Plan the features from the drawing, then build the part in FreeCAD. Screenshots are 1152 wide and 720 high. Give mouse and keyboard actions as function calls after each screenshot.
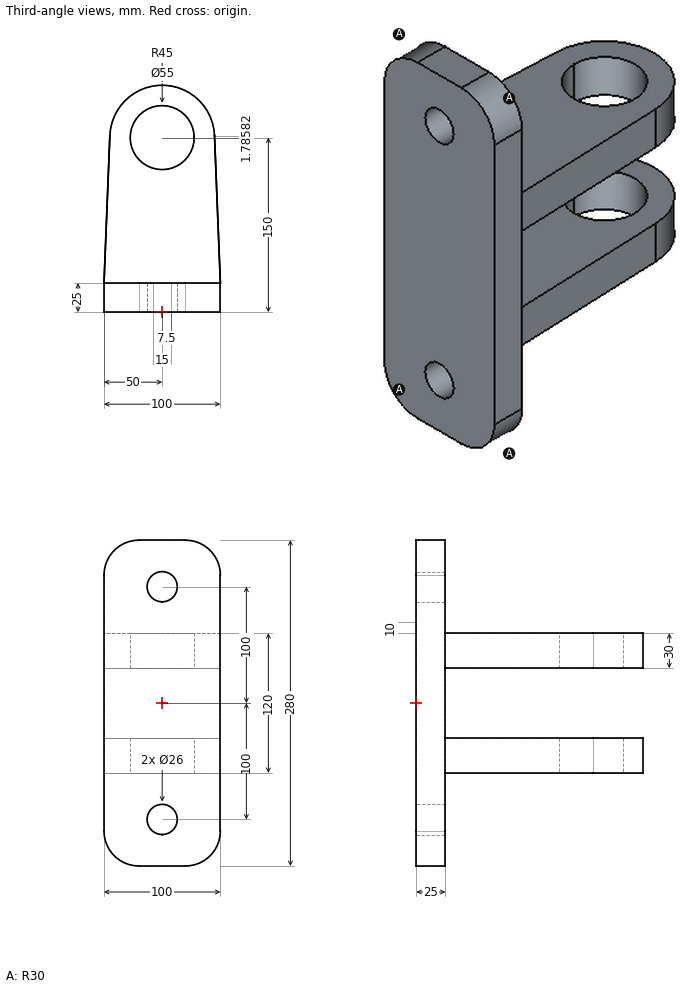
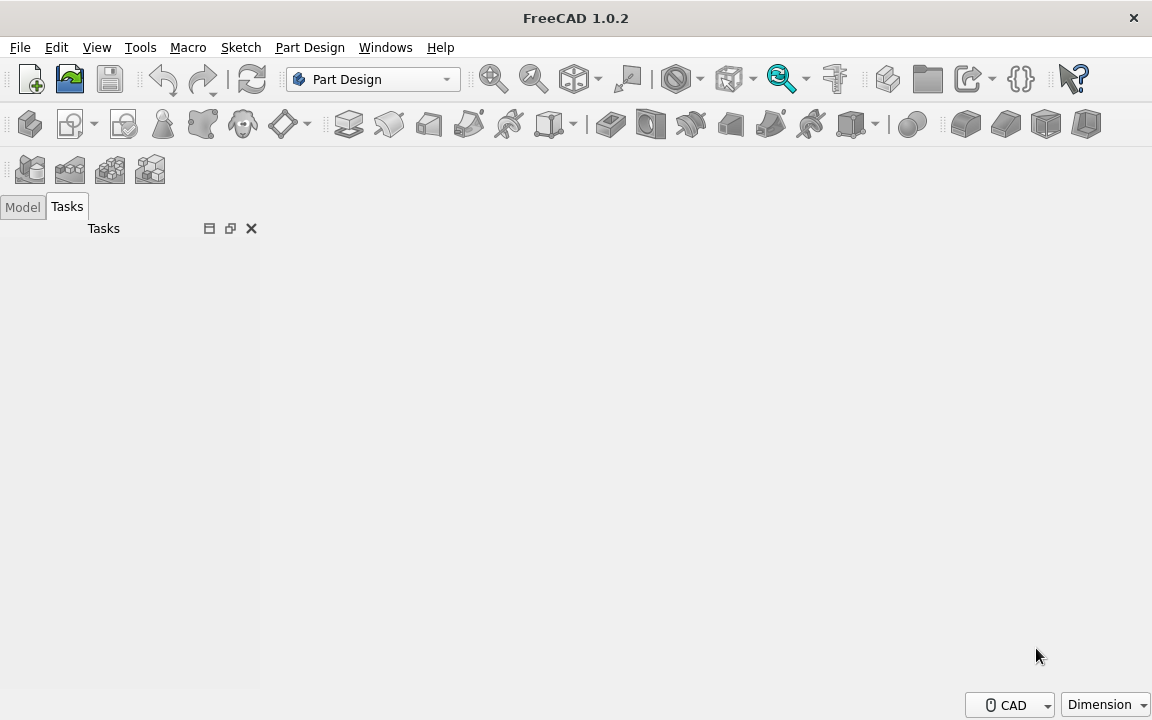
click(30, 80)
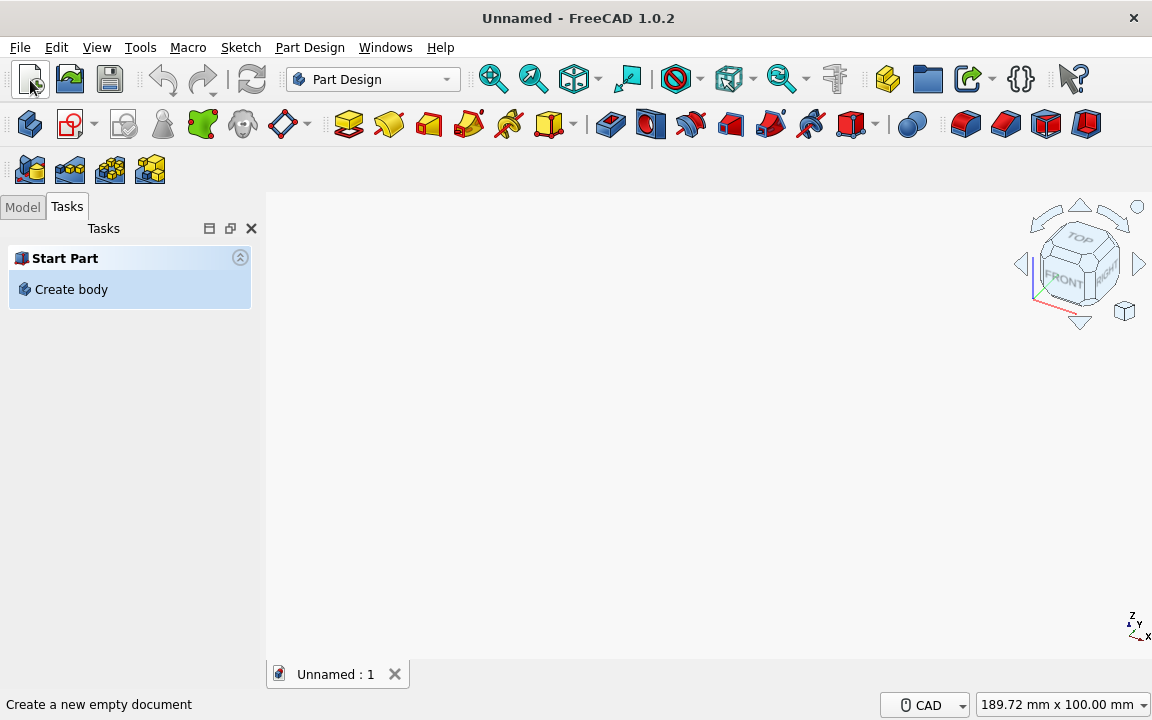
click(70, 124)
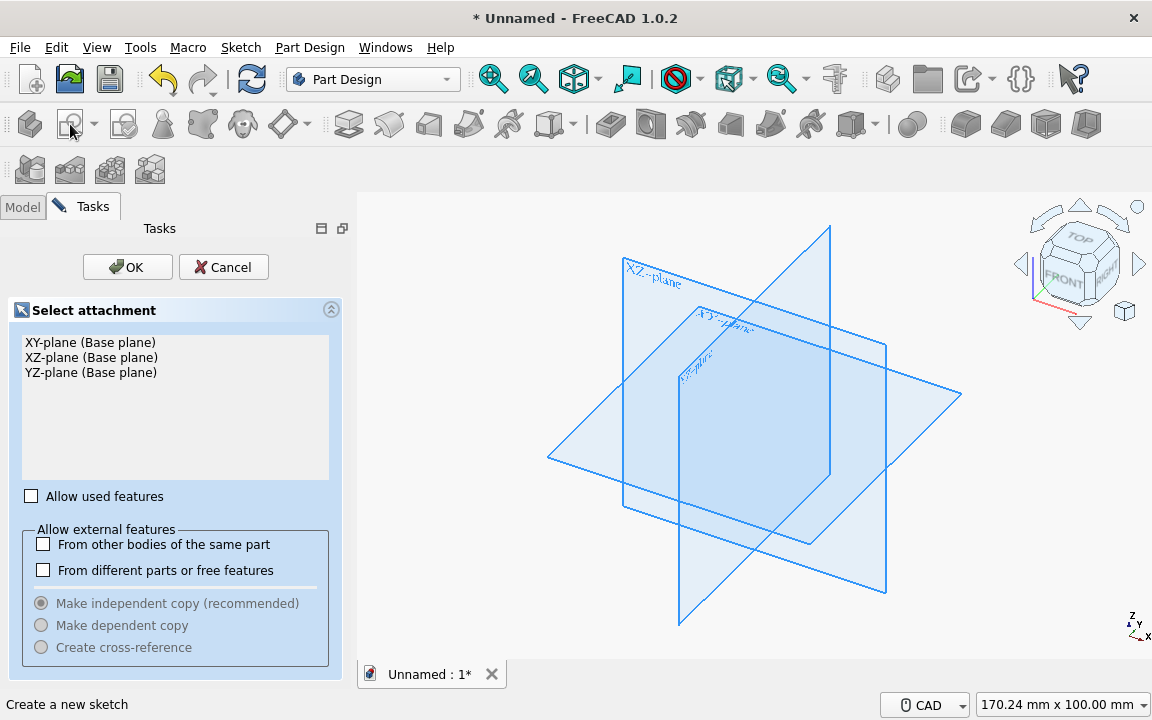
click(82, 358)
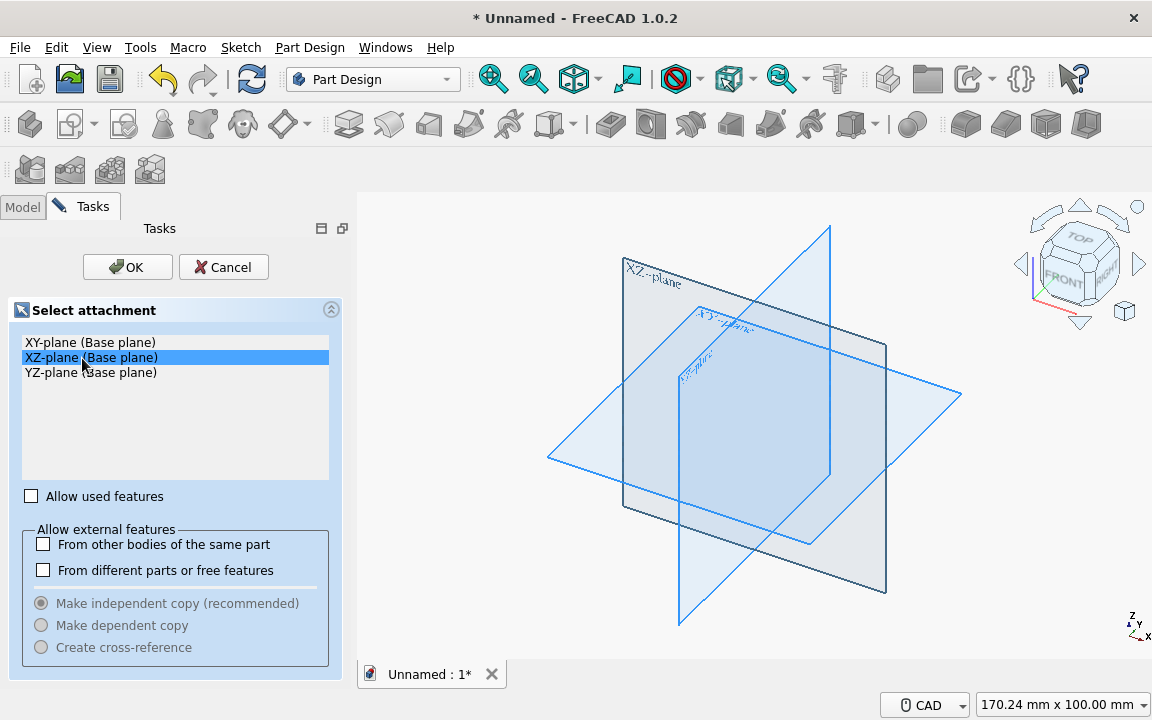
click(128, 267)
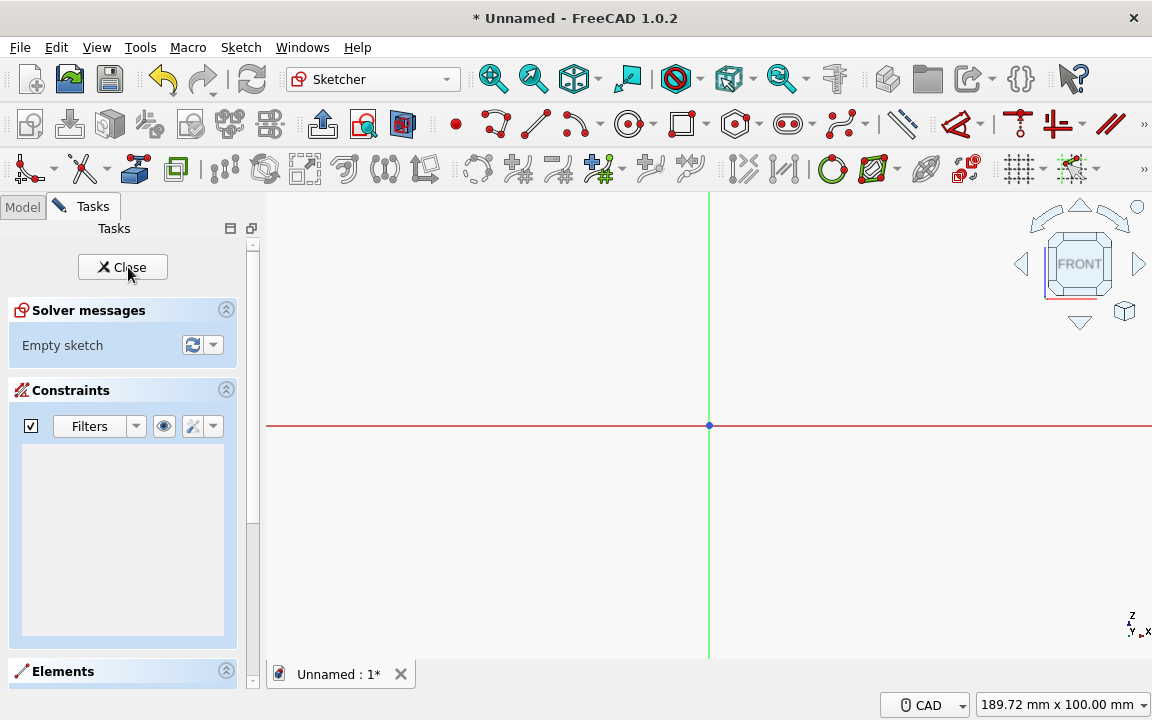
scroll(557, 426, down, 3)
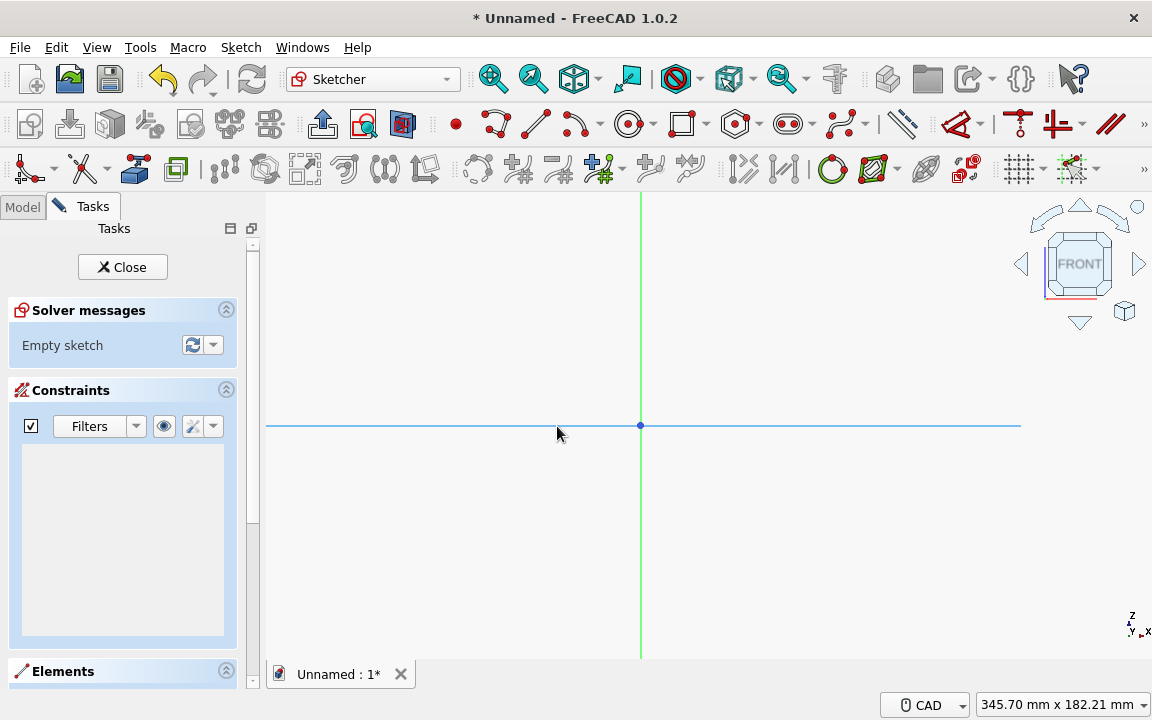
key(g)
key(v)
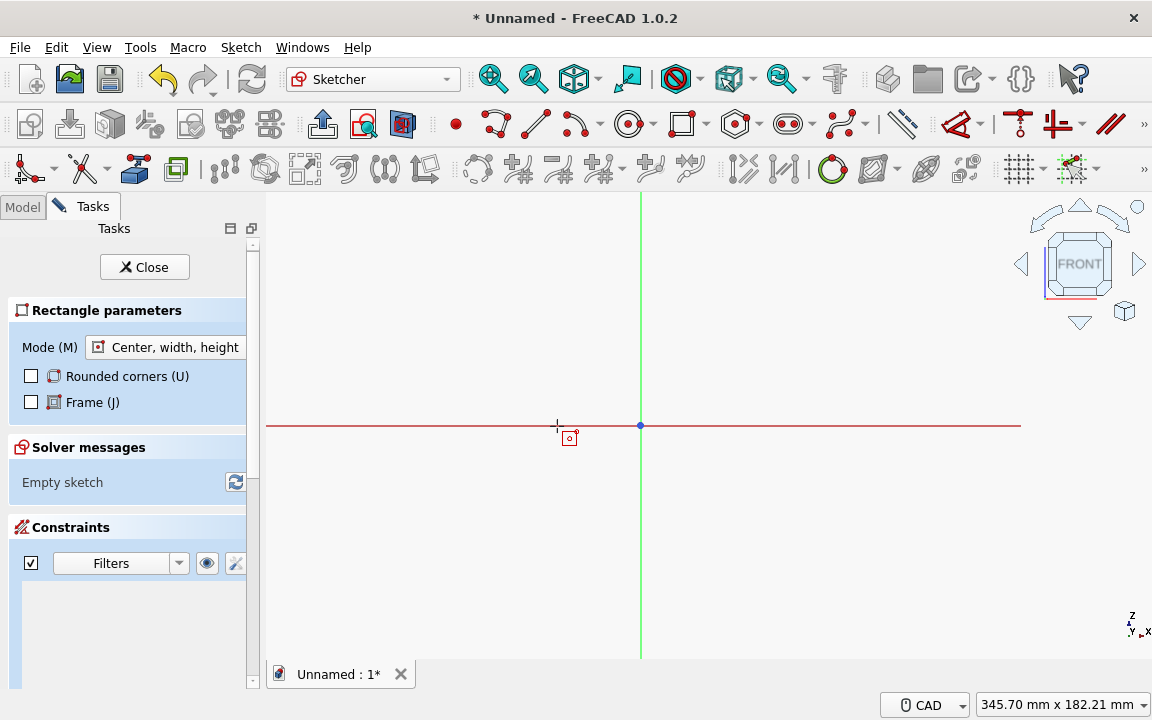
click(641, 426)
click(769, 272)
key(Escape)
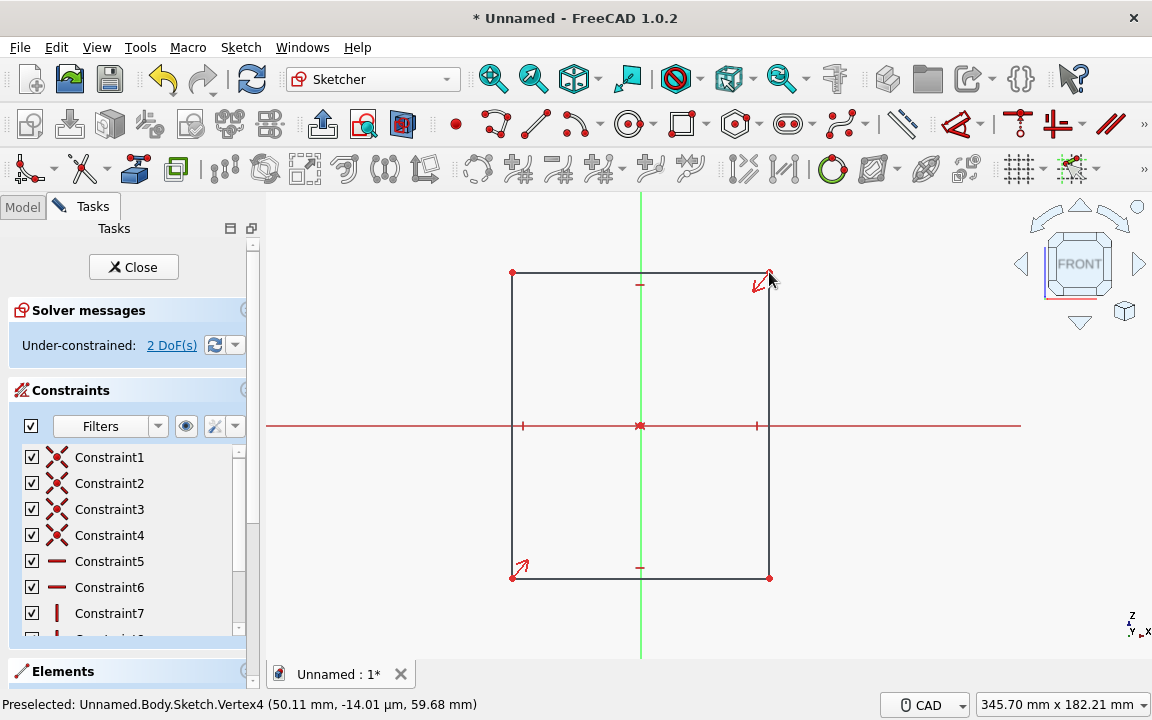
click(589, 579)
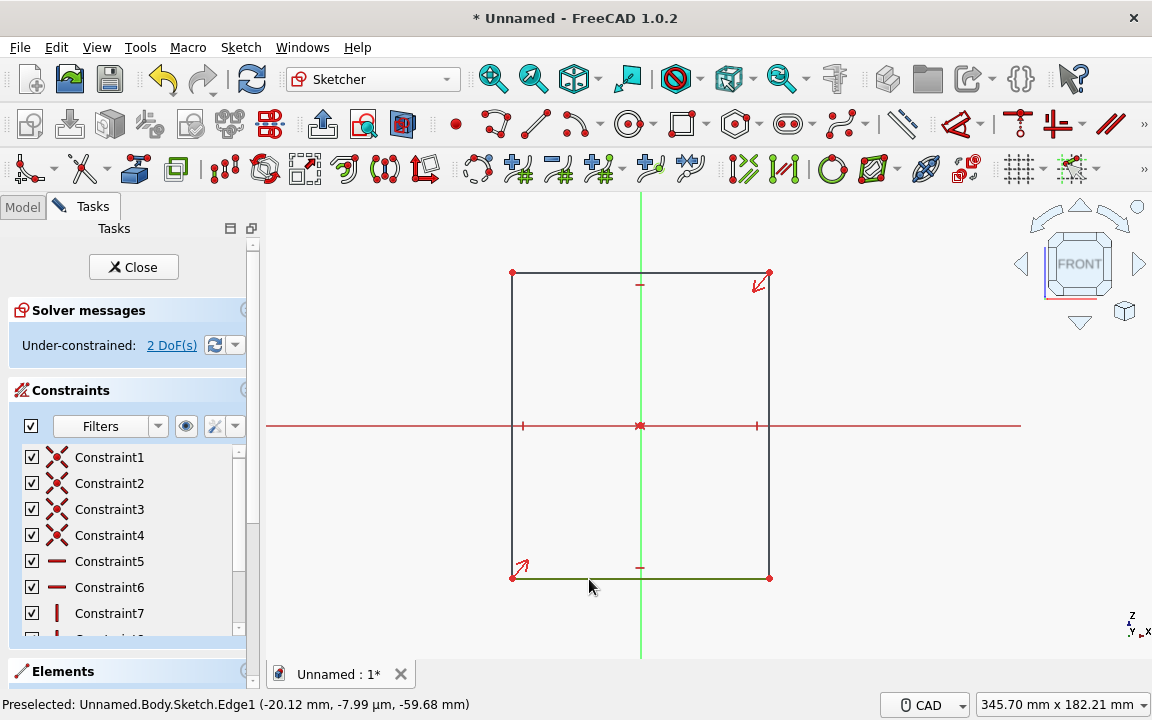
key(l)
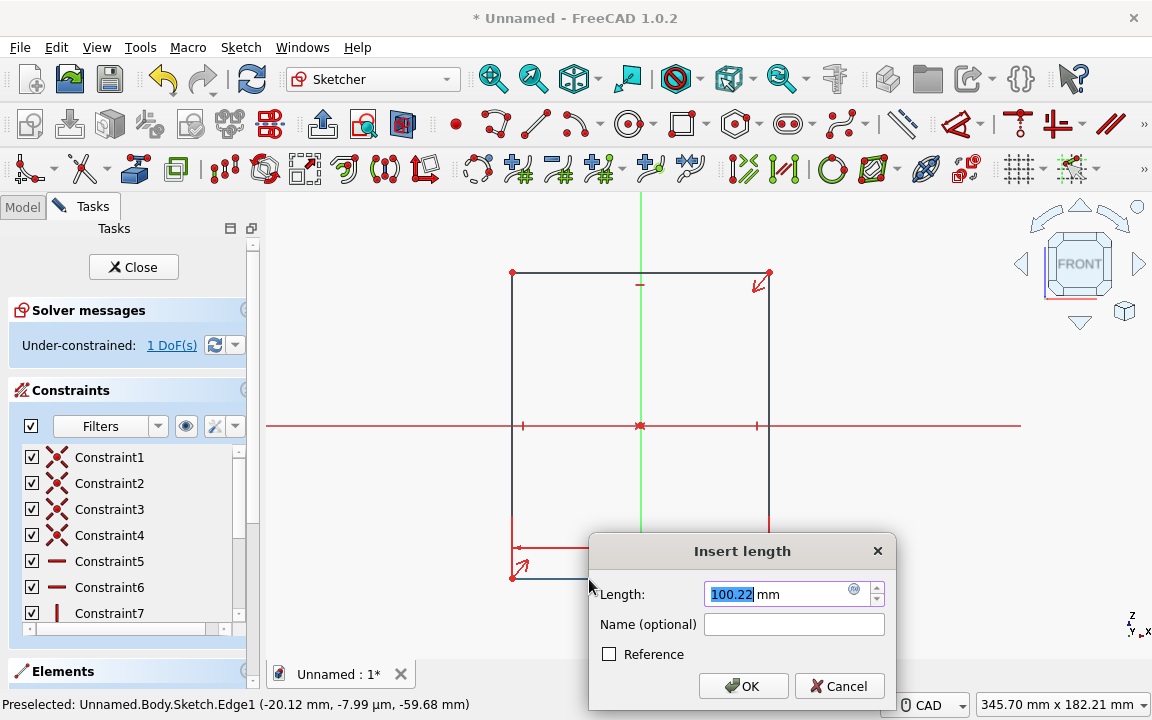
text(100)
key(Return)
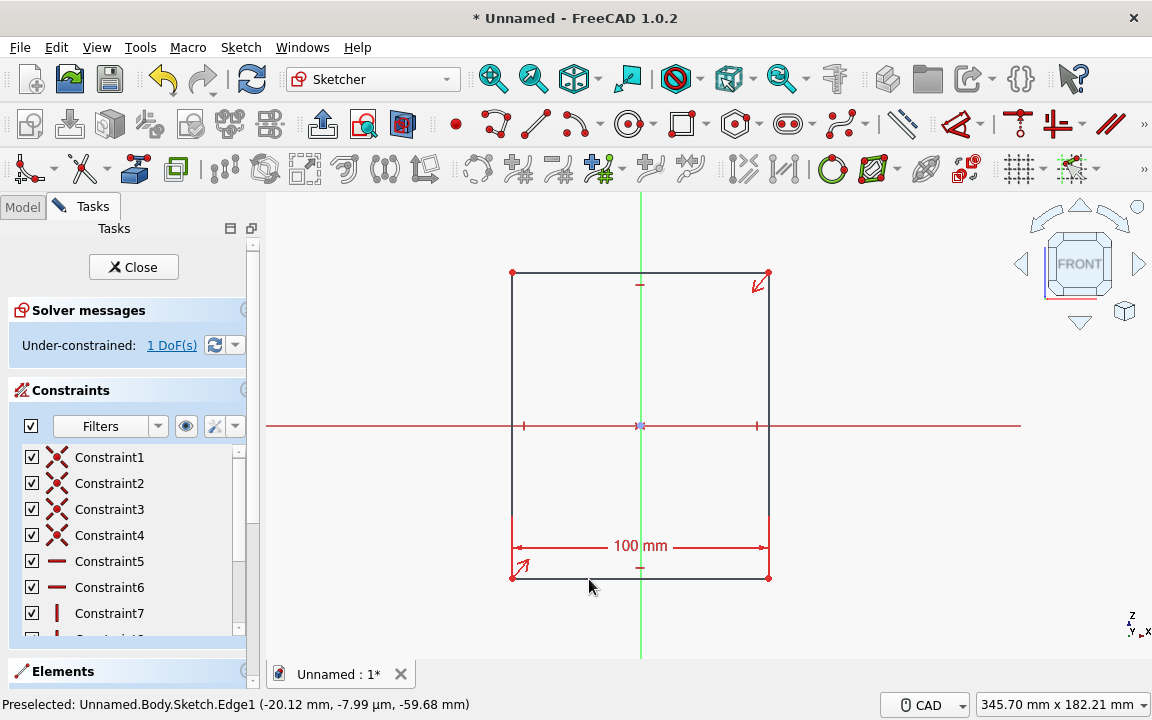
click(769, 487)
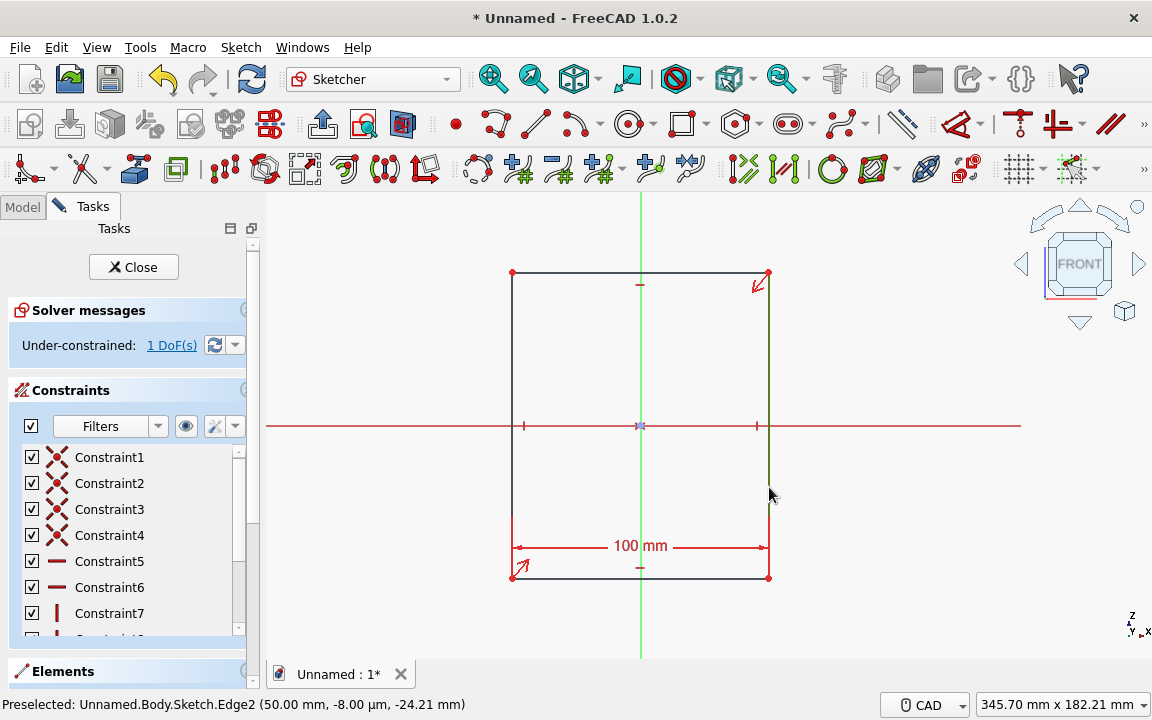
click(982, 124)